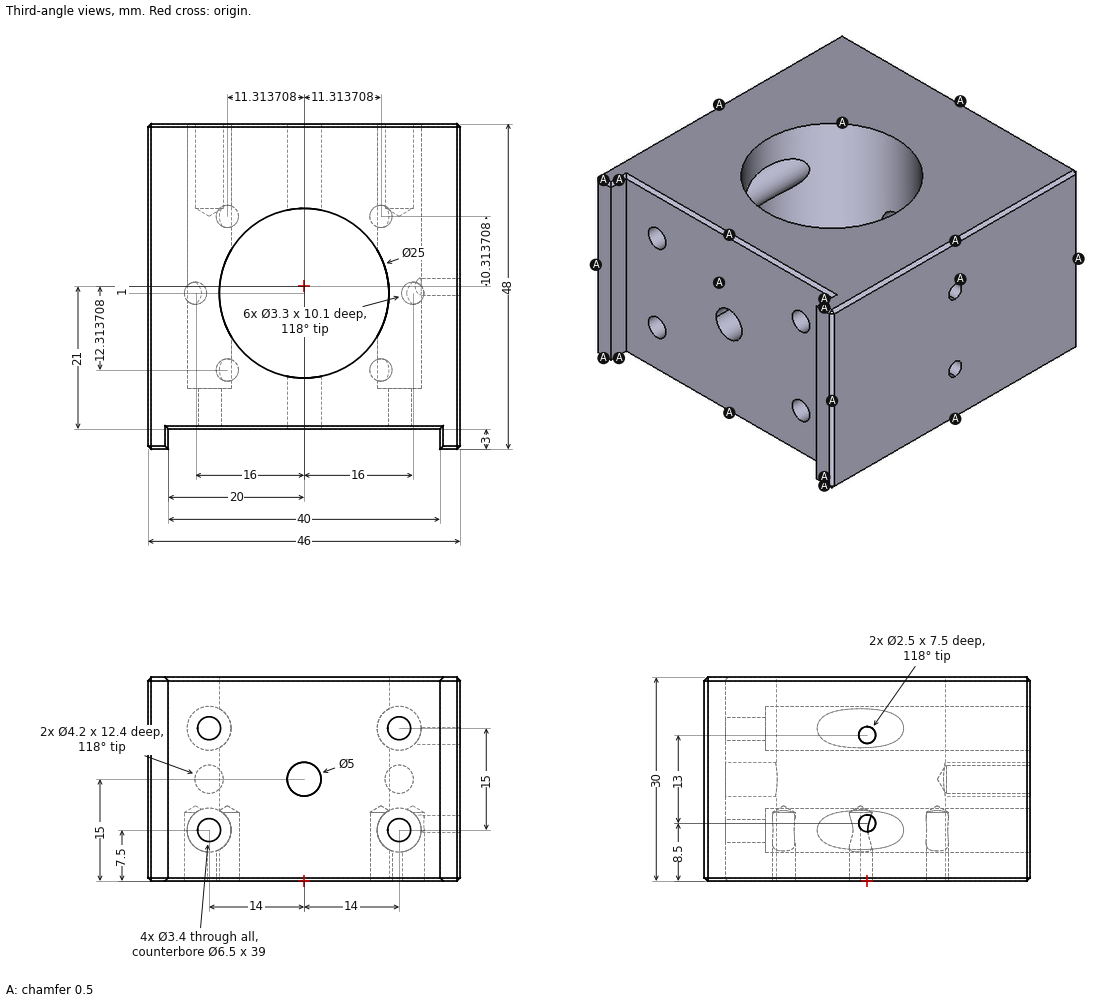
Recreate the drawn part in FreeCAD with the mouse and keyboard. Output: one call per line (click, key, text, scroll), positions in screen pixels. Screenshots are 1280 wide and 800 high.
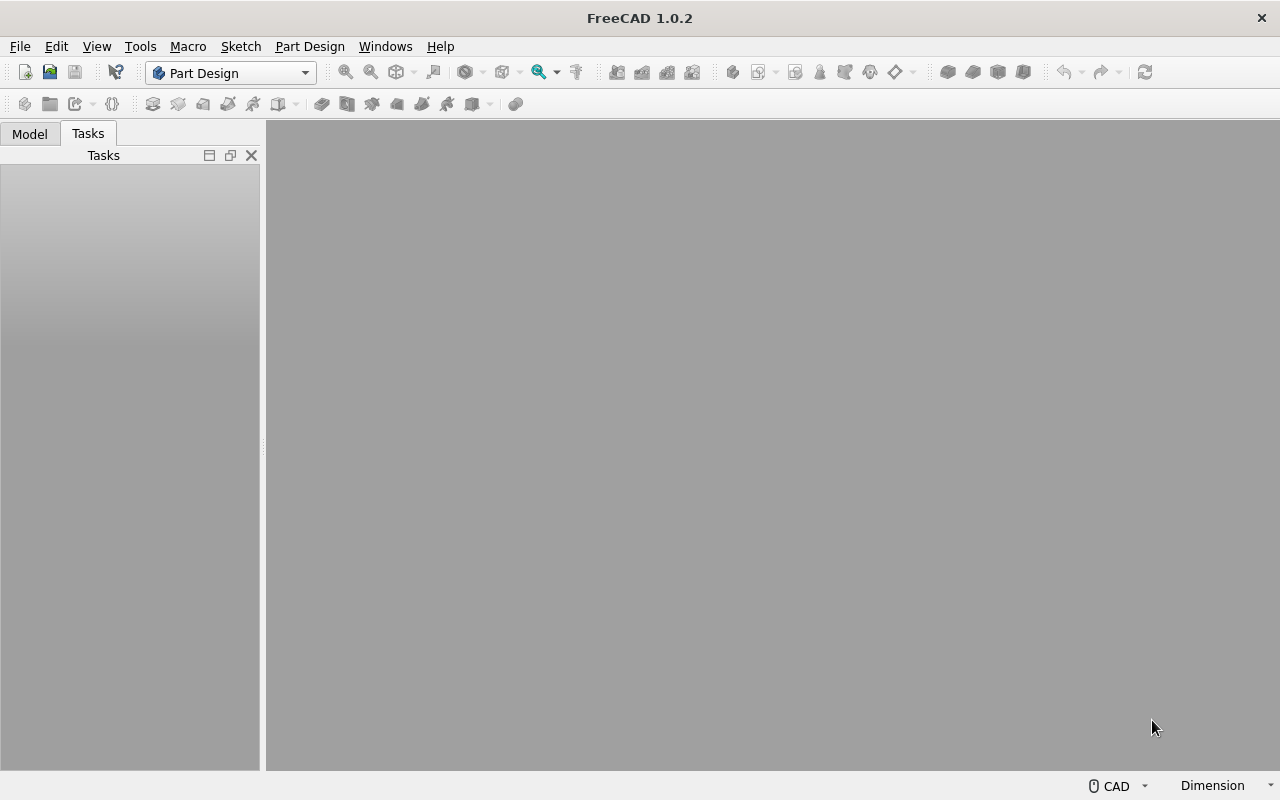
click(25, 72)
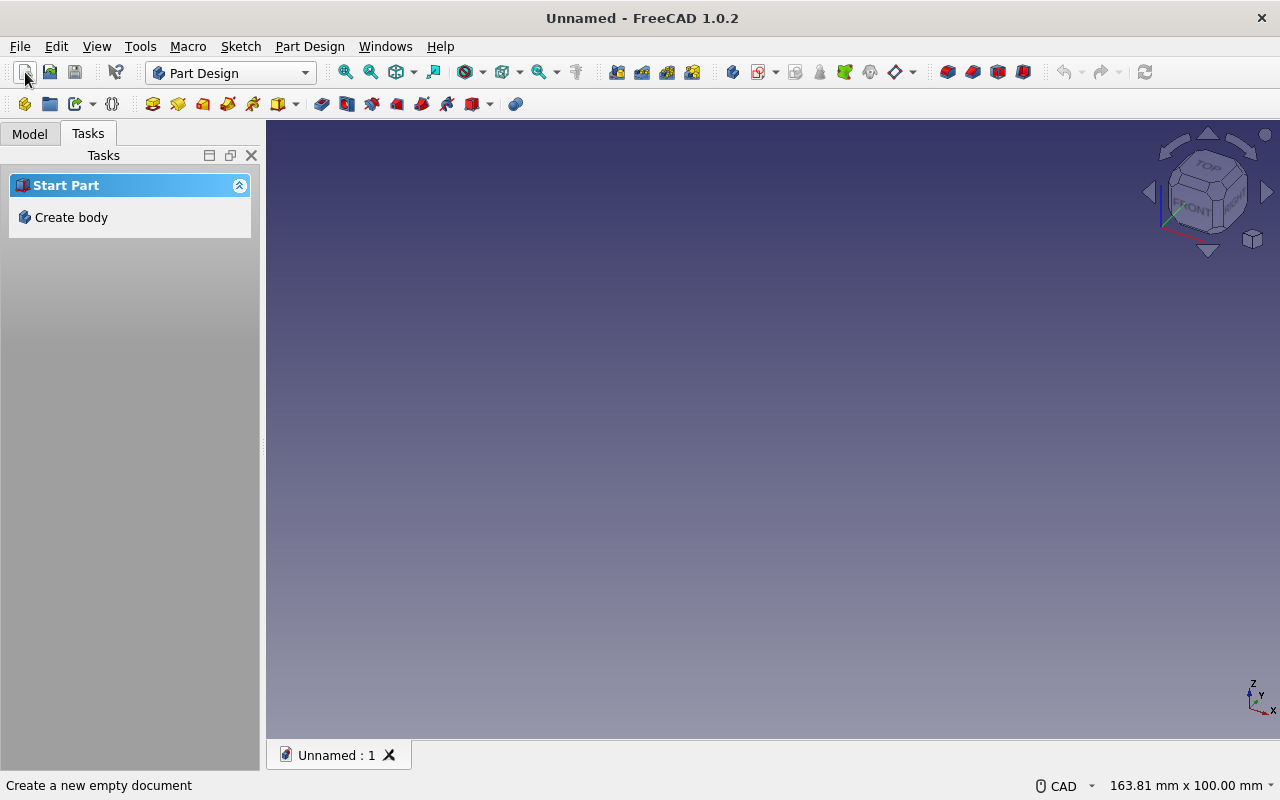
click(758, 72)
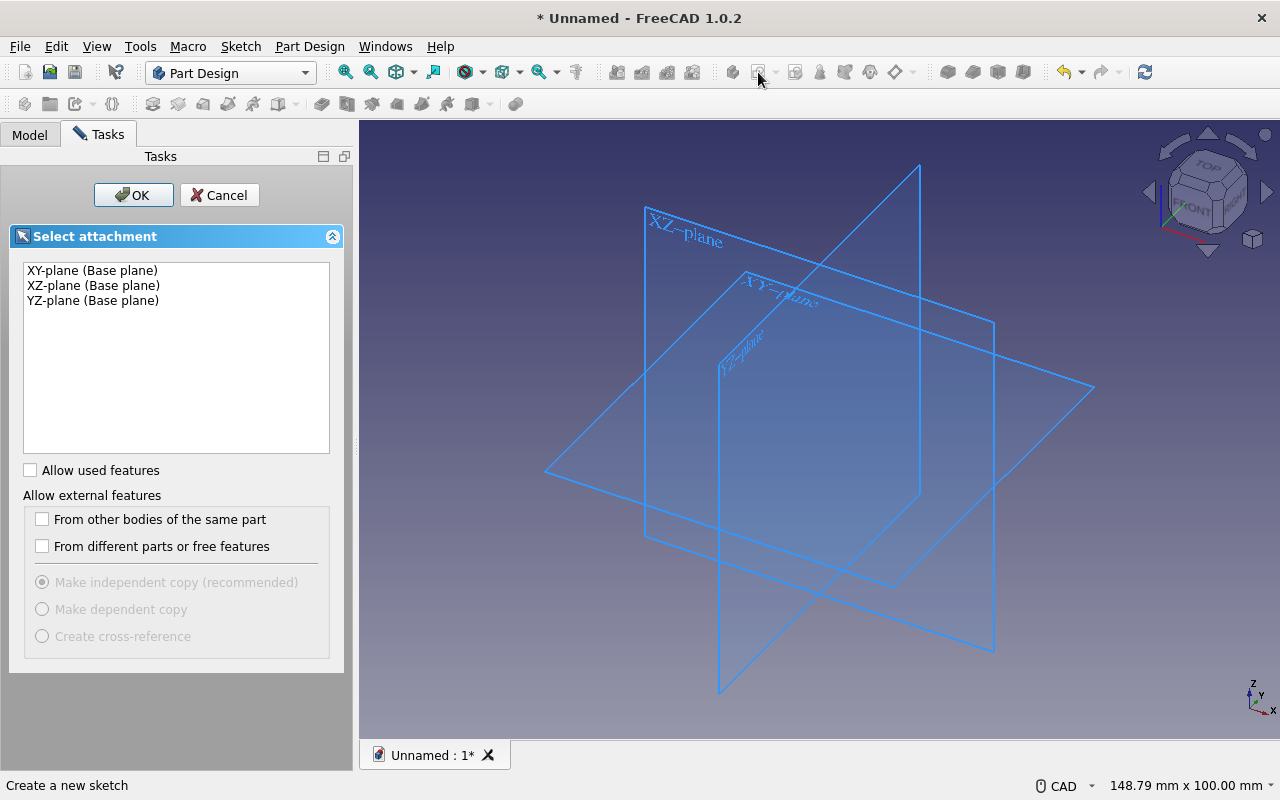
click(84, 270)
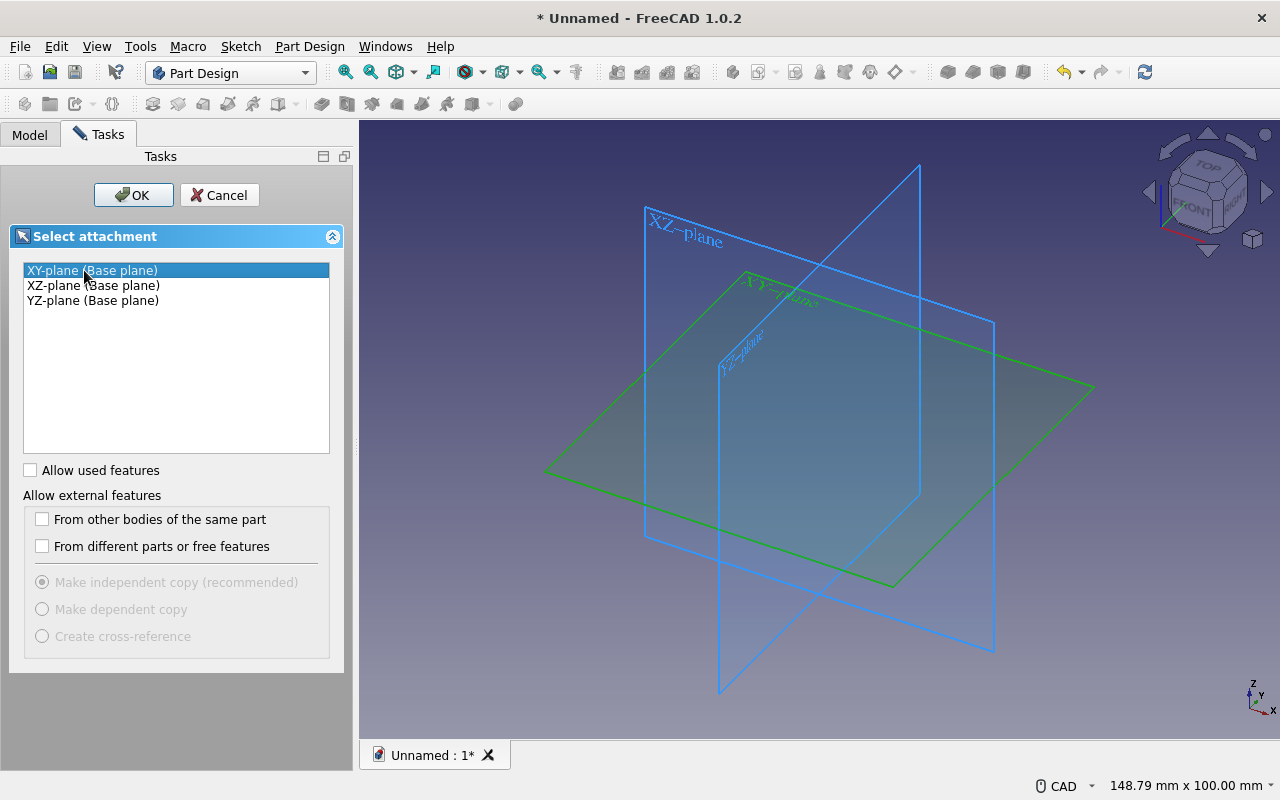
click(134, 195)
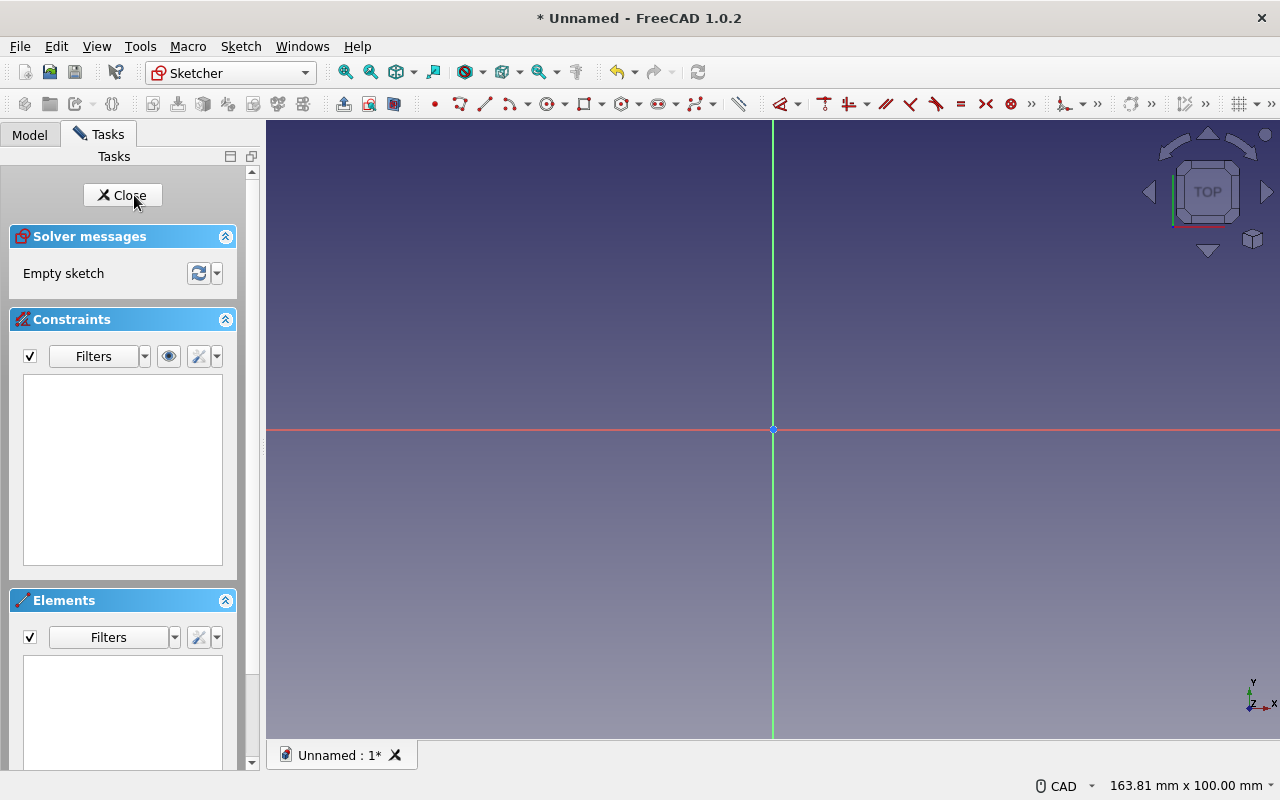
click(602, 104)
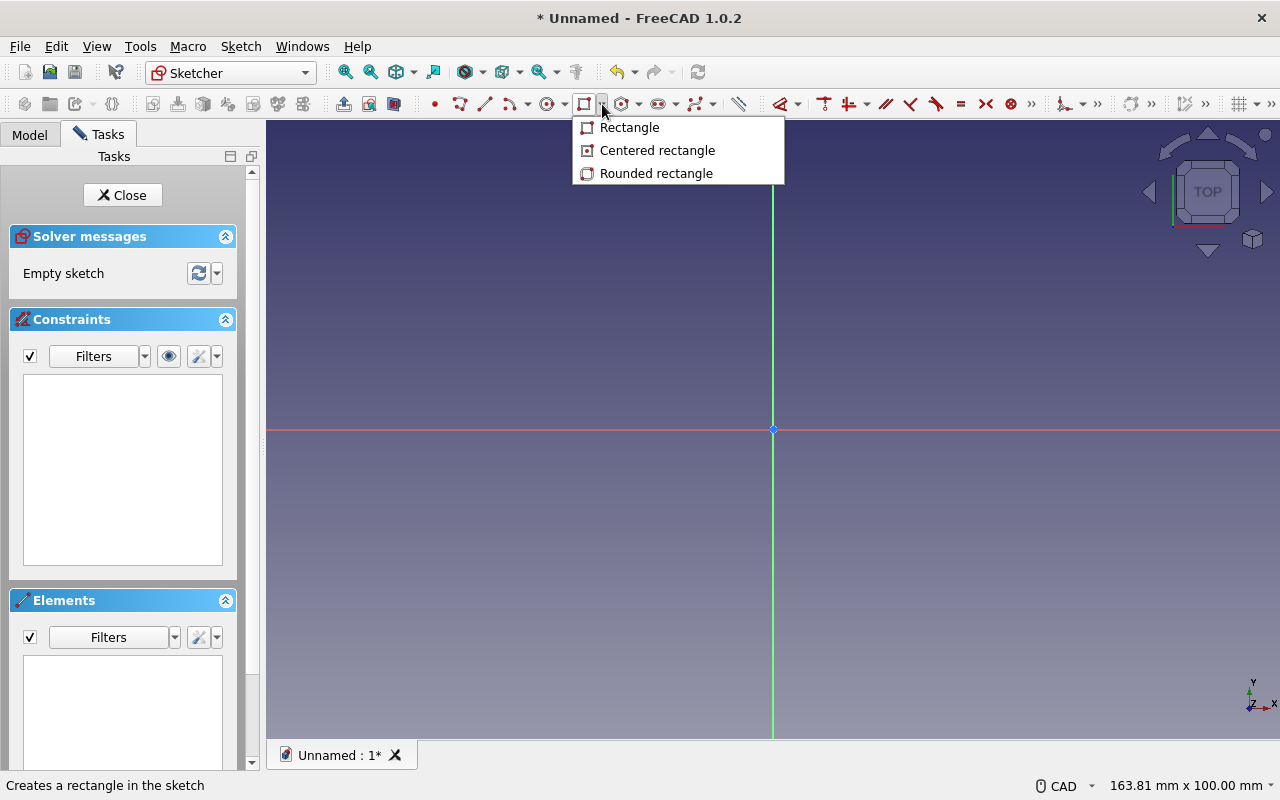
click(678, 150)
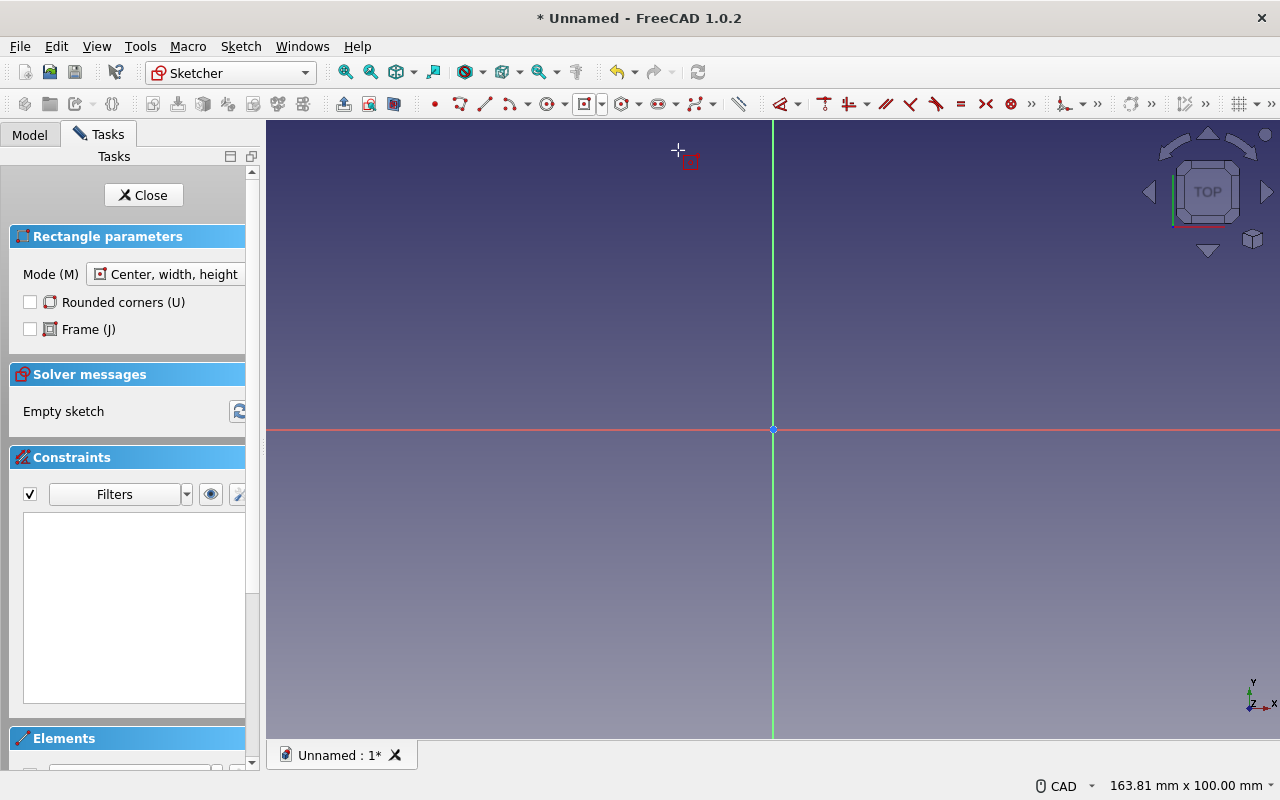
click(773, 430)
move(915, 281)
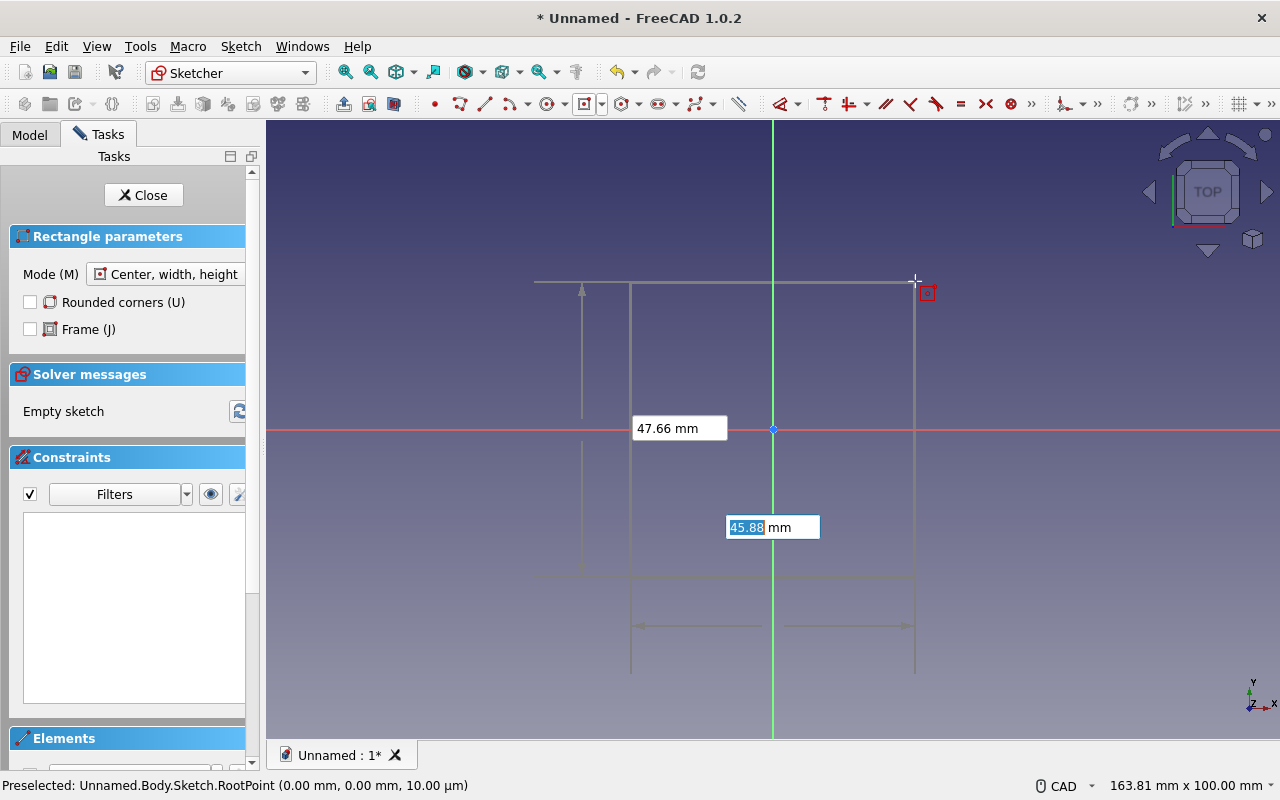
text(46)
key(Tab)
text(48)
key(Return)
key(Escape)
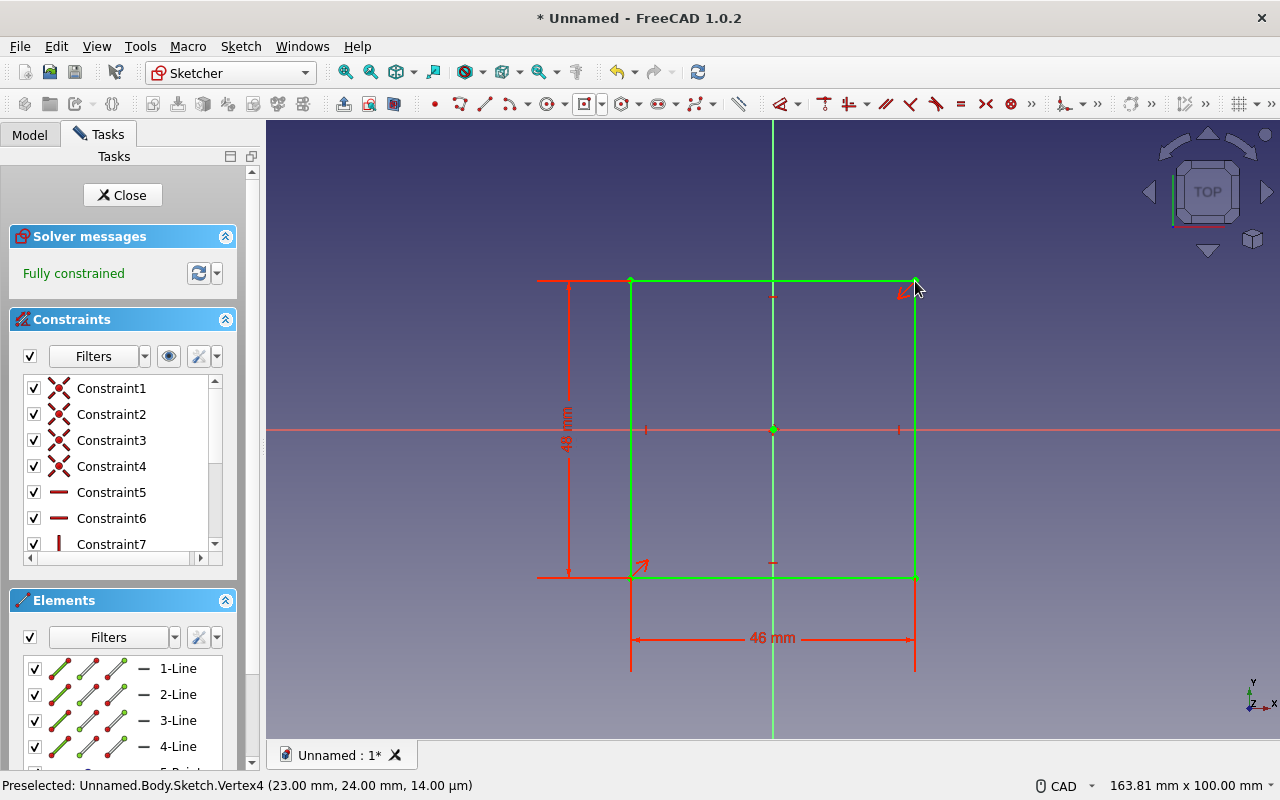
click(123, 195)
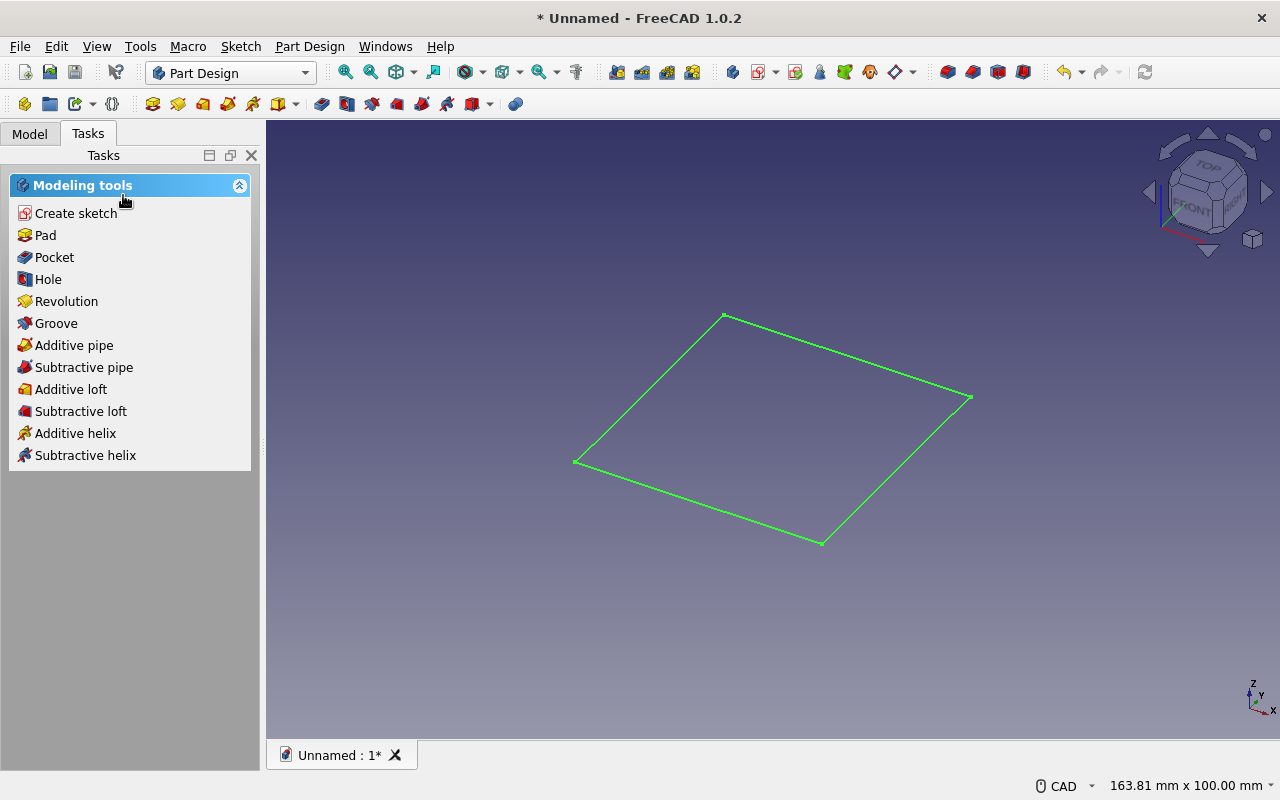
click(153, 104)